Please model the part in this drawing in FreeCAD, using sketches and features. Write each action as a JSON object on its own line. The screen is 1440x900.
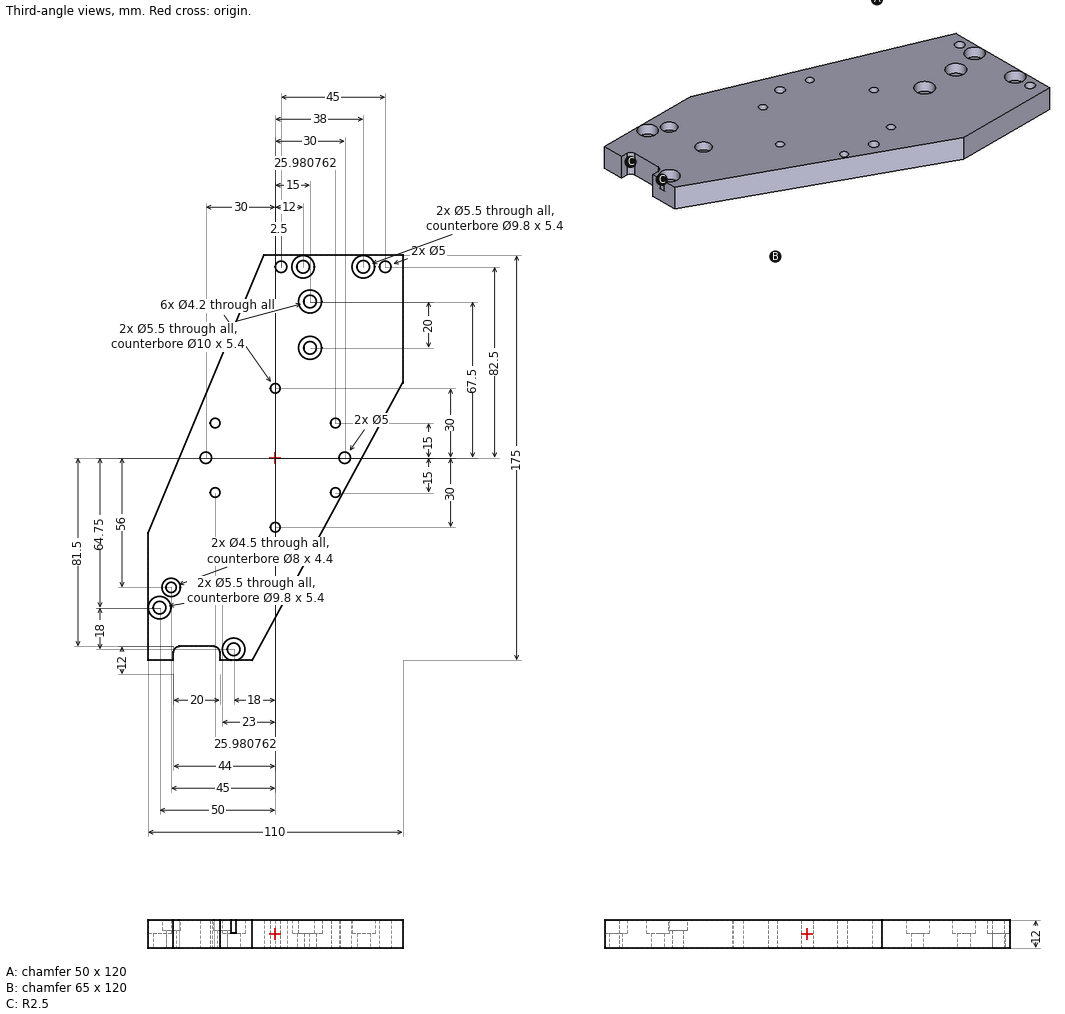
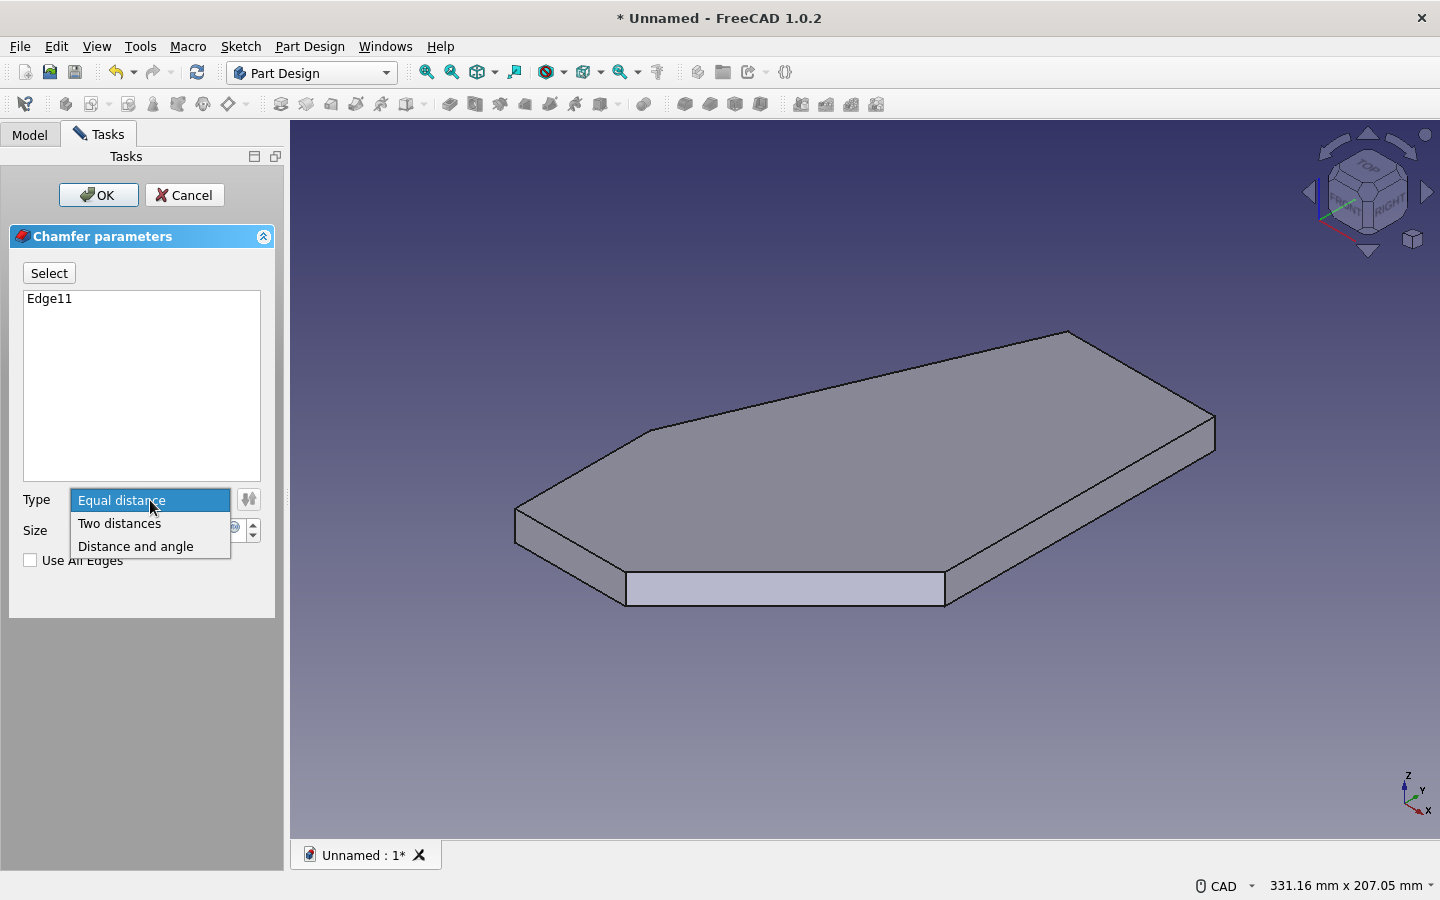
{"action": "left_click", "coordinate": [148, 524]}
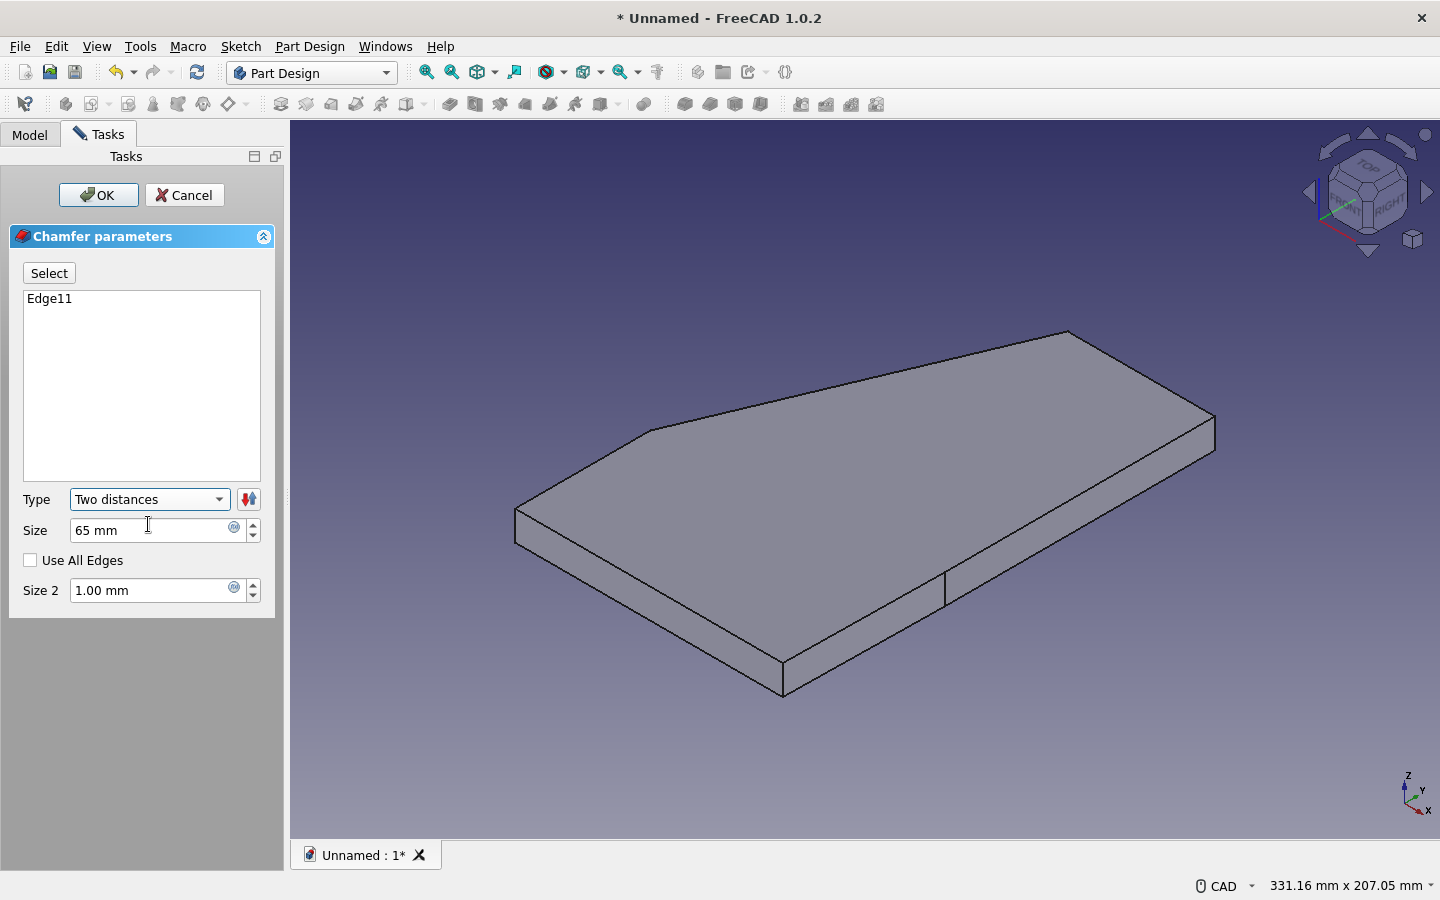
{"action": "triple_click", "coordinate": [158, 590]}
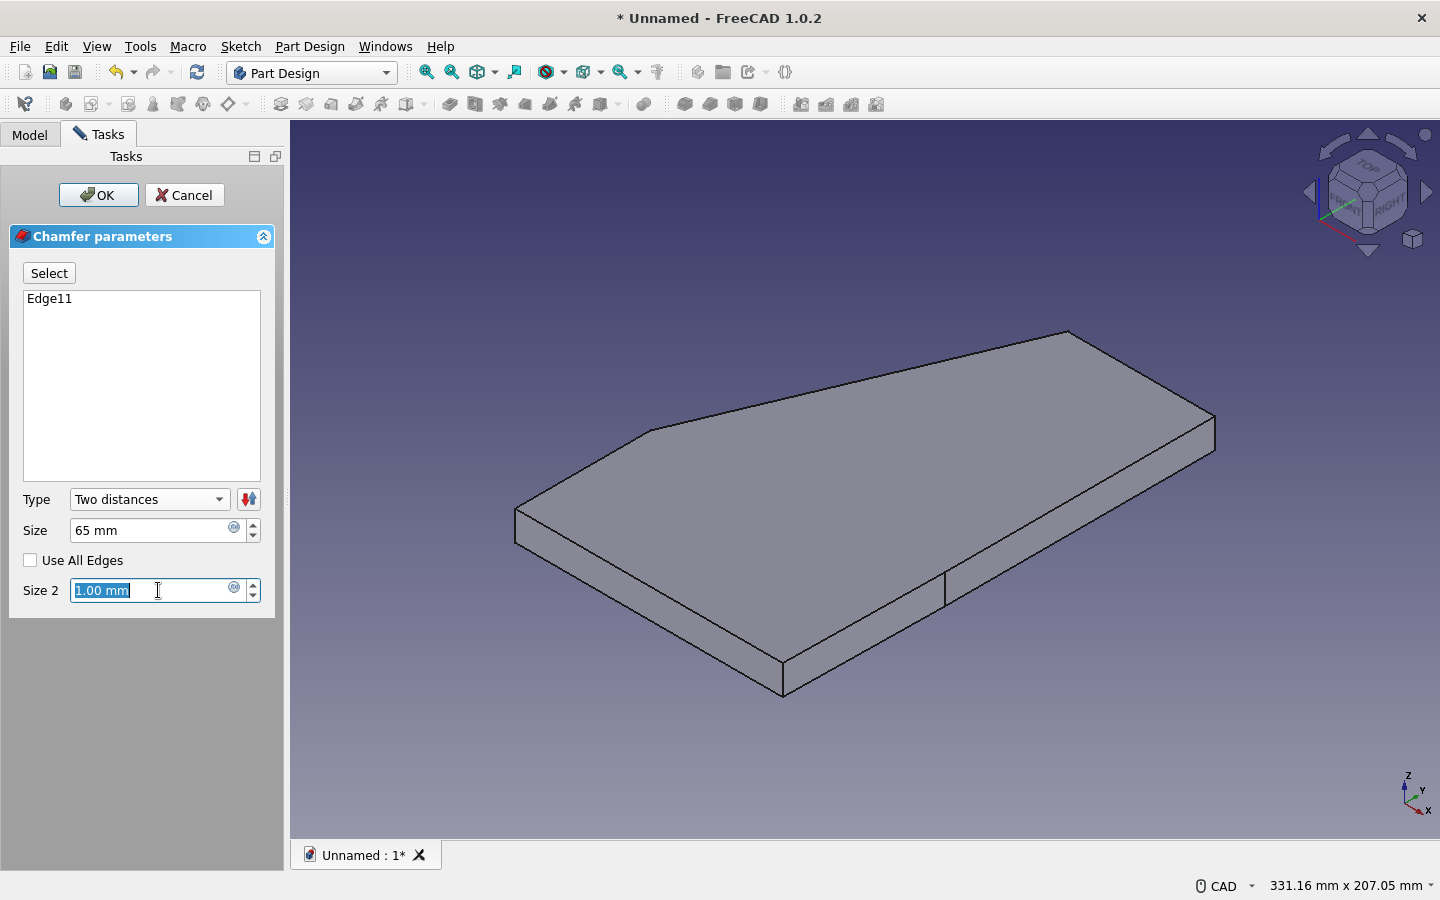
{"action": "type", "text": "120"}
{"action": "key", "text": "Tab"}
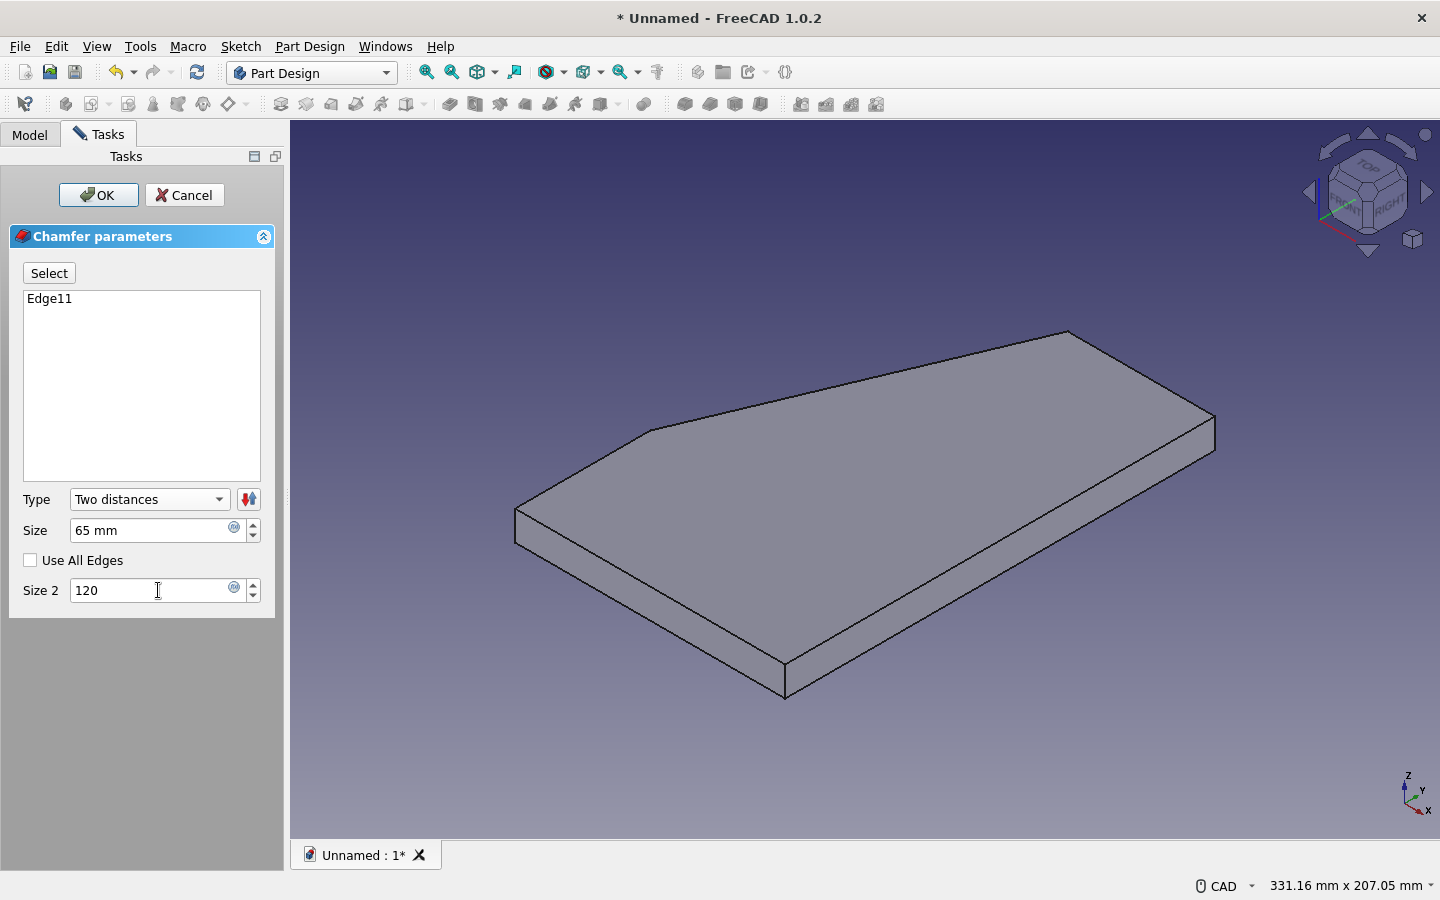
{"action": "left_click", "coordinate": [249, 500]}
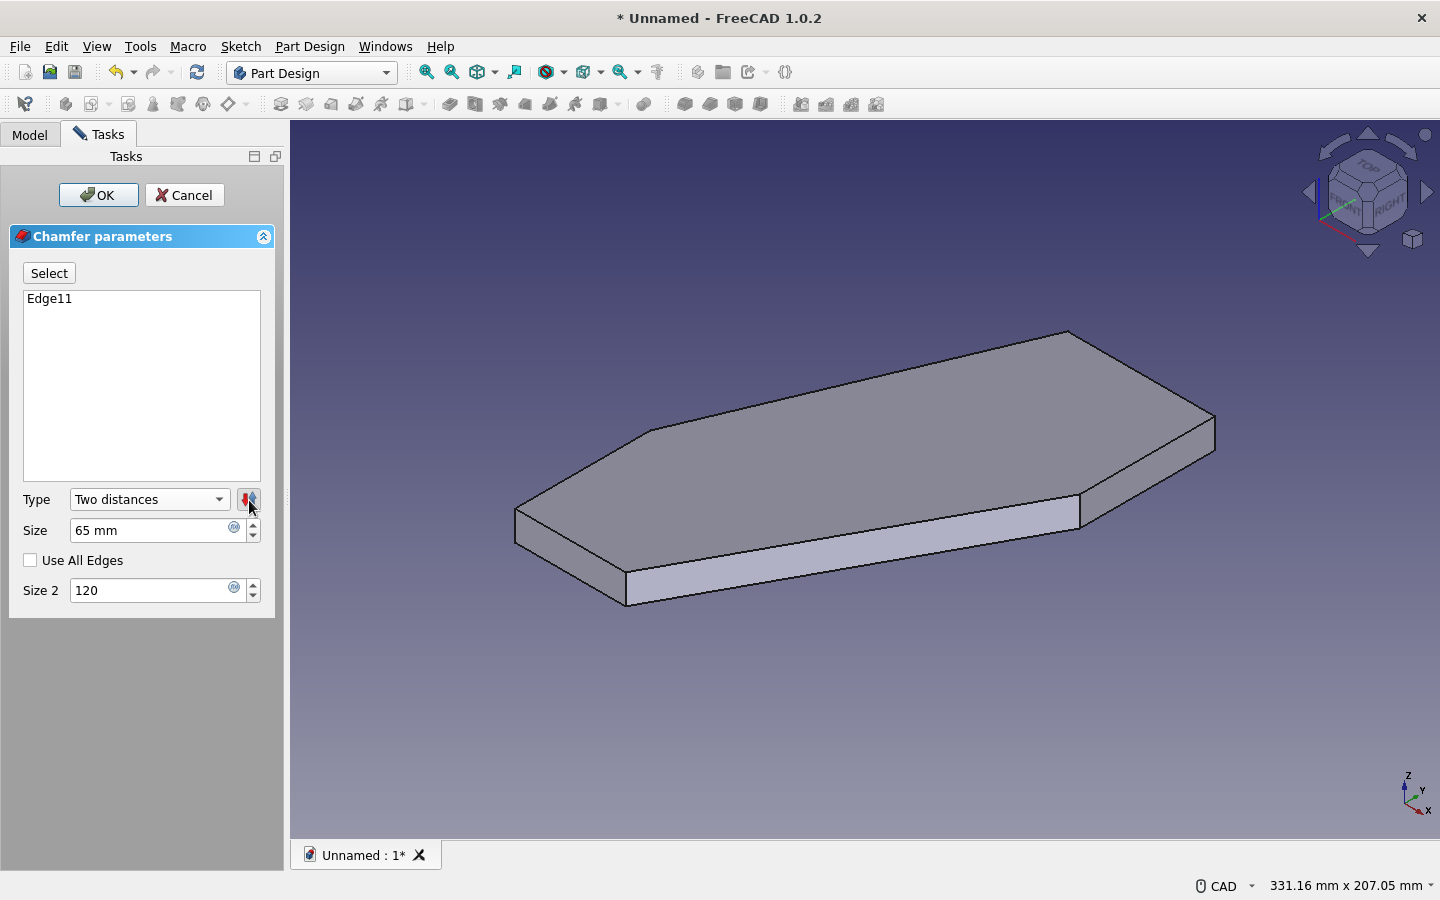
{"action": "left_click", "coordinate": [99, 195]}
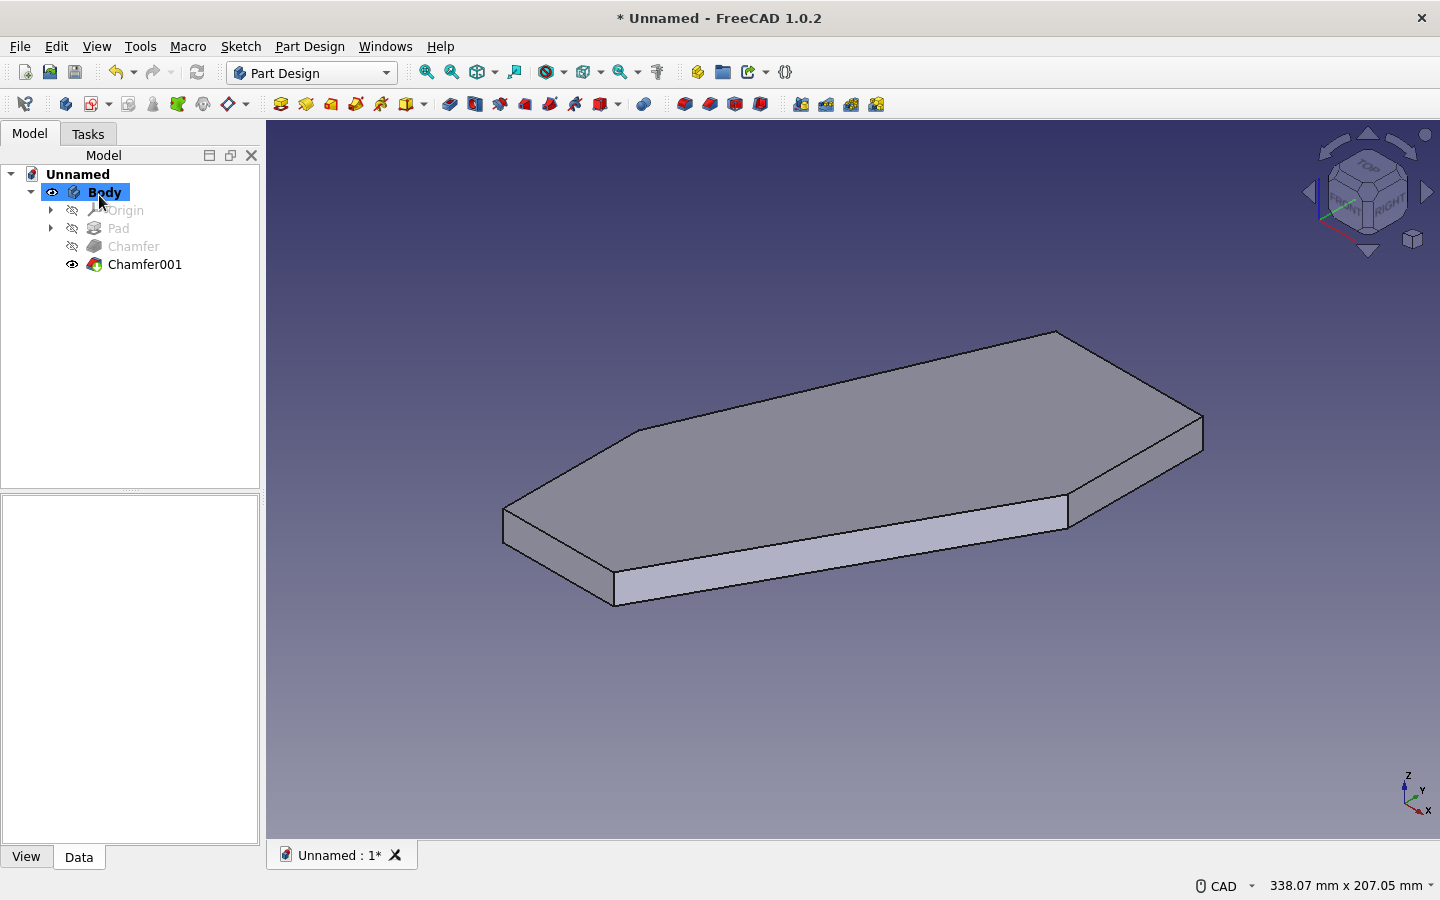
{"action": "left_click", "coordinate": [1014, 413]}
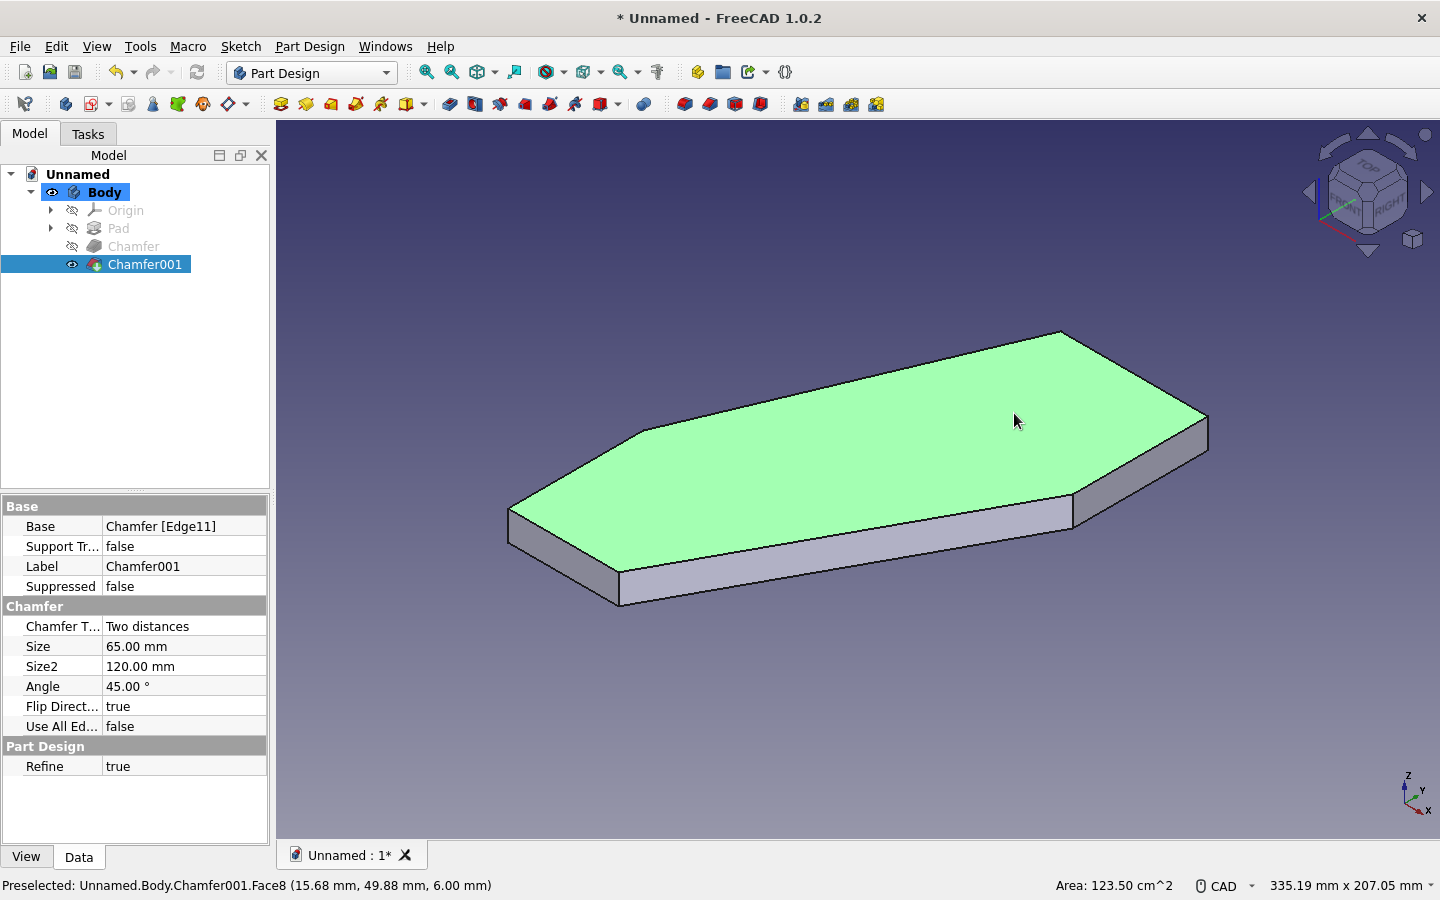
{"action": "left_click", "coordinate": [90, 104]}